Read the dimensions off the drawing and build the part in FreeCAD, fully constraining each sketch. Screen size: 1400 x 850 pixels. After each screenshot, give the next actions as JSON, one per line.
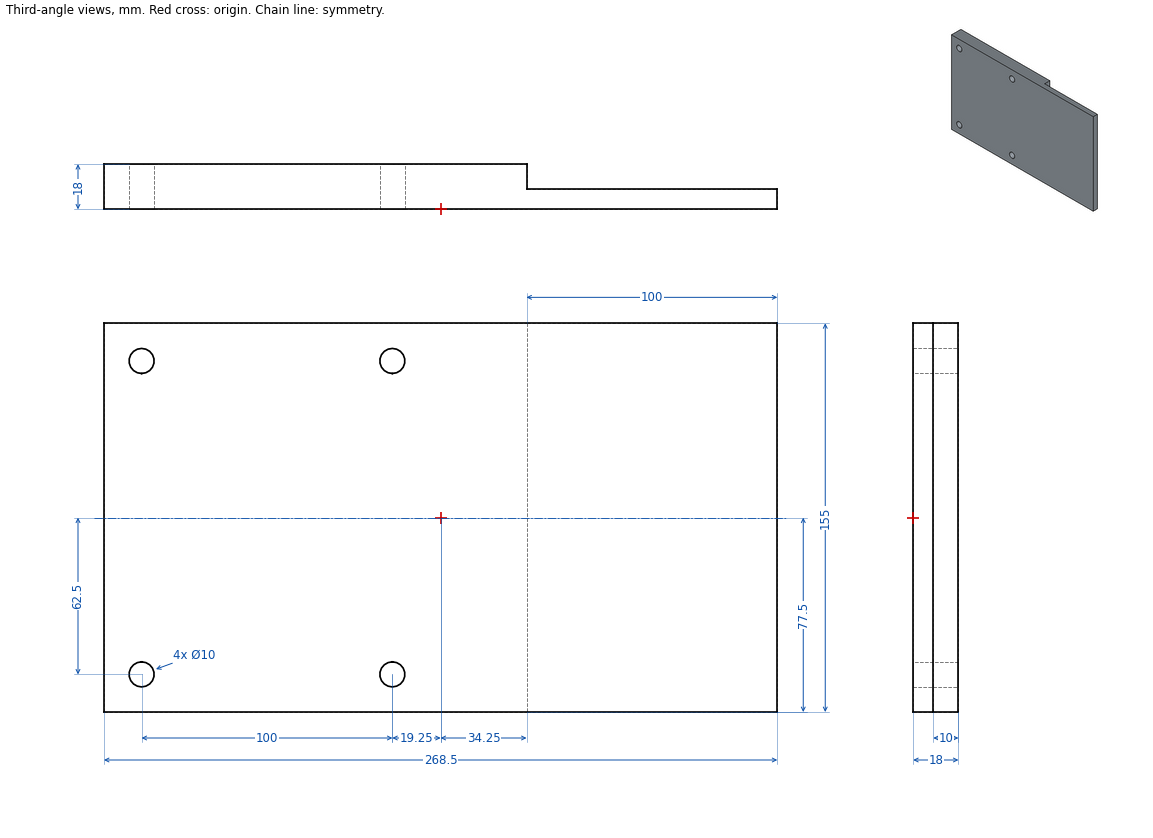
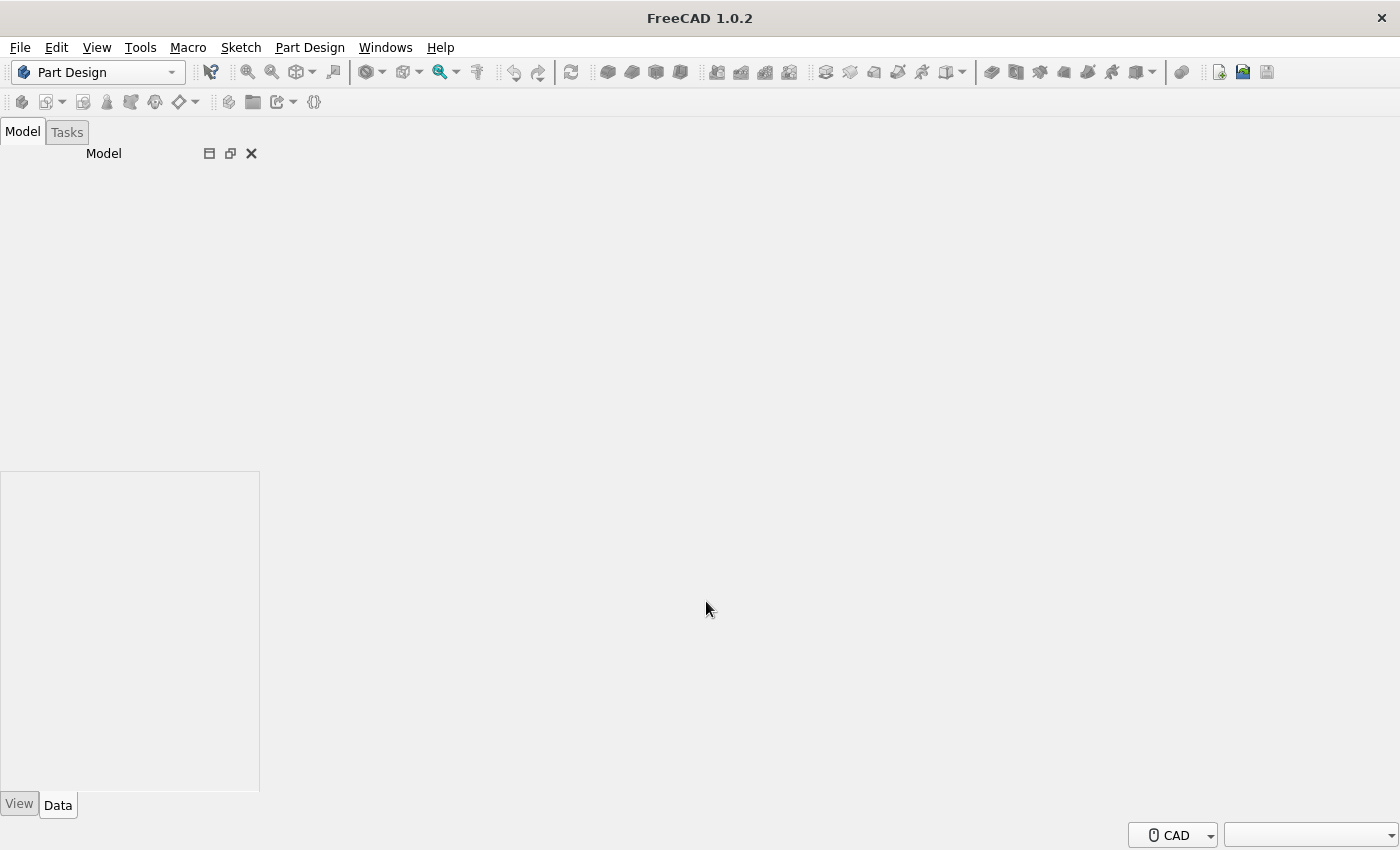
{"action": "left_click", "coordinate": [1220, 72]}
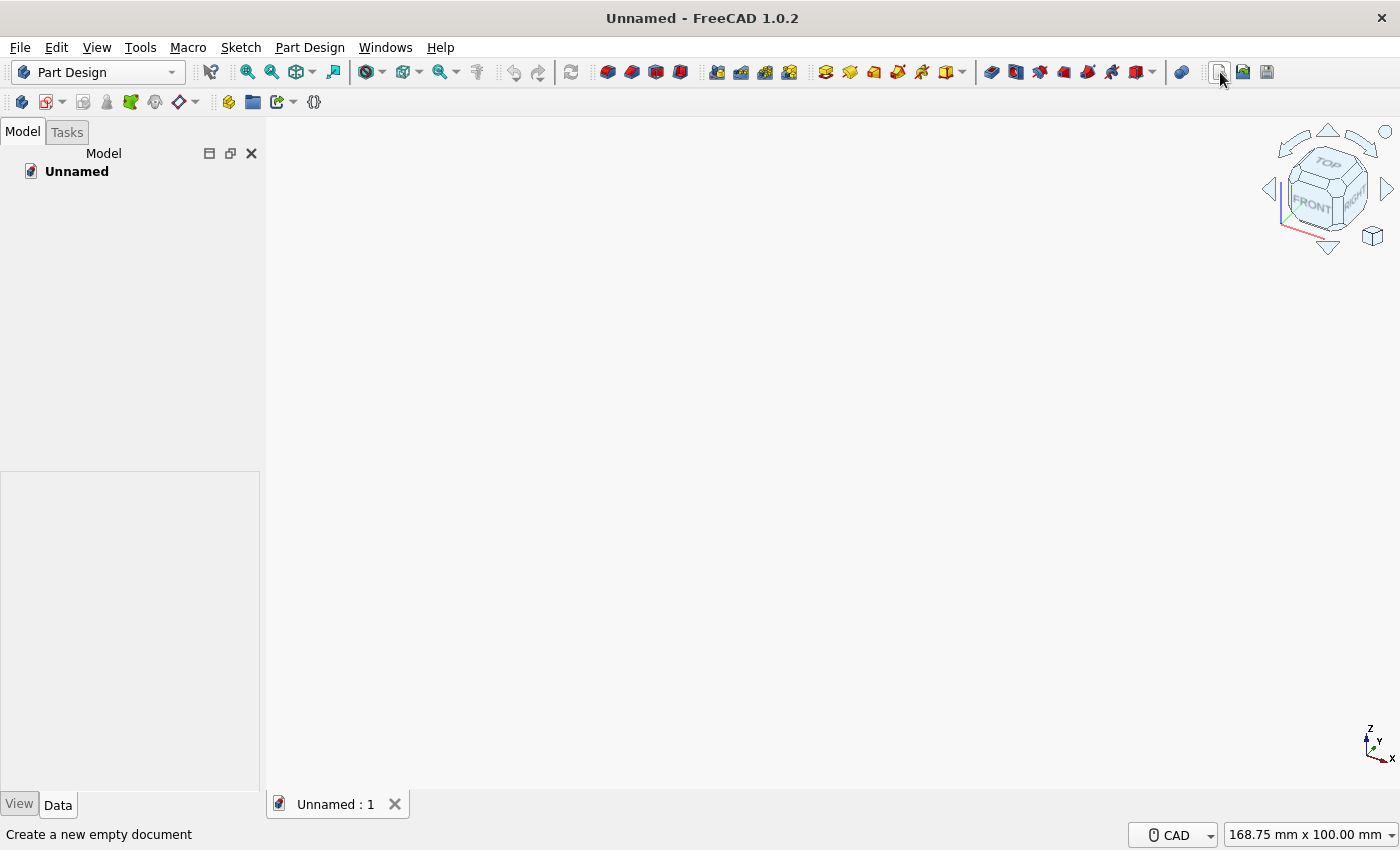
{"action": "left_click", "coordinate": [46, 102]}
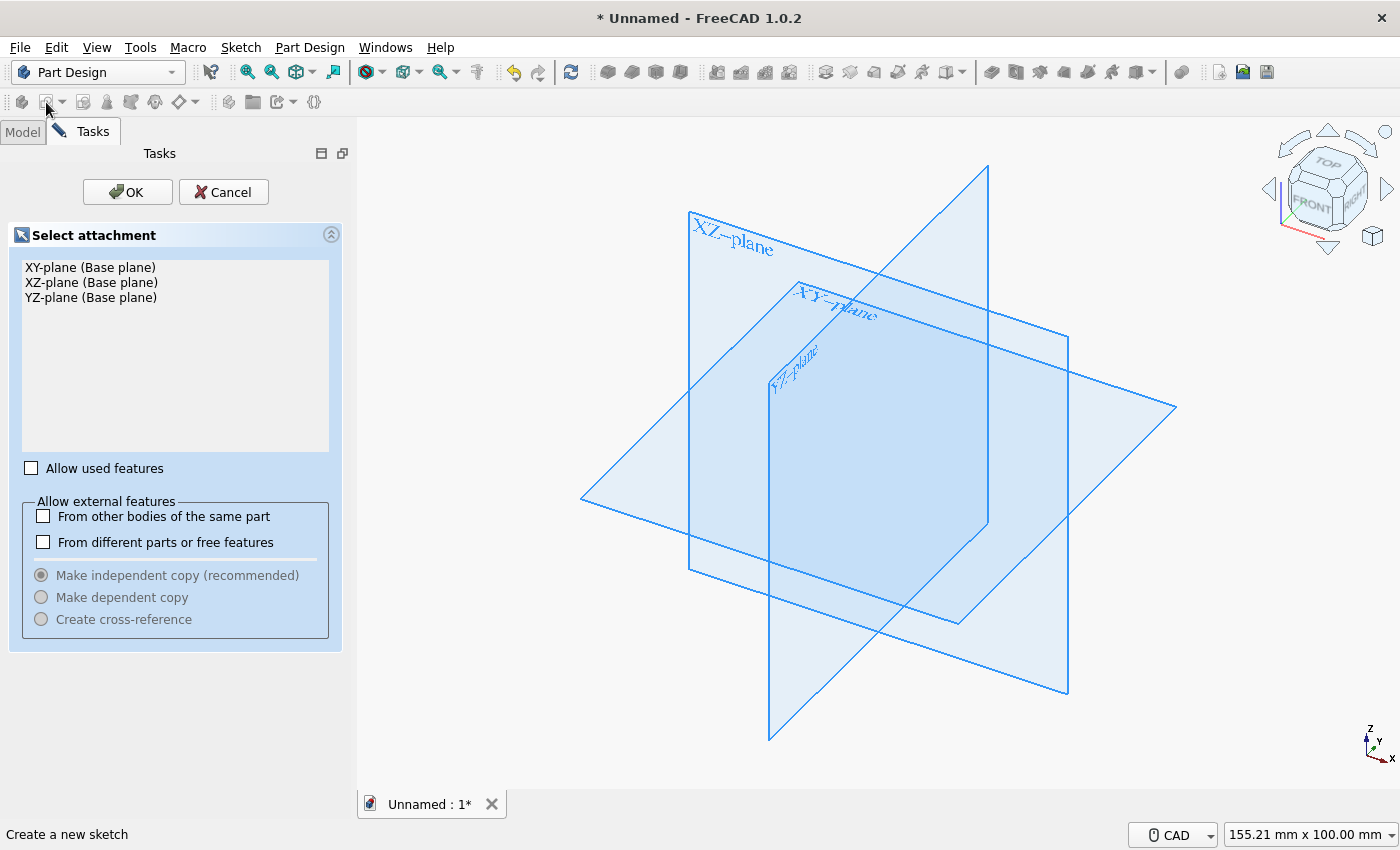
{"action": "left_click", "coordinate": [82, 282]}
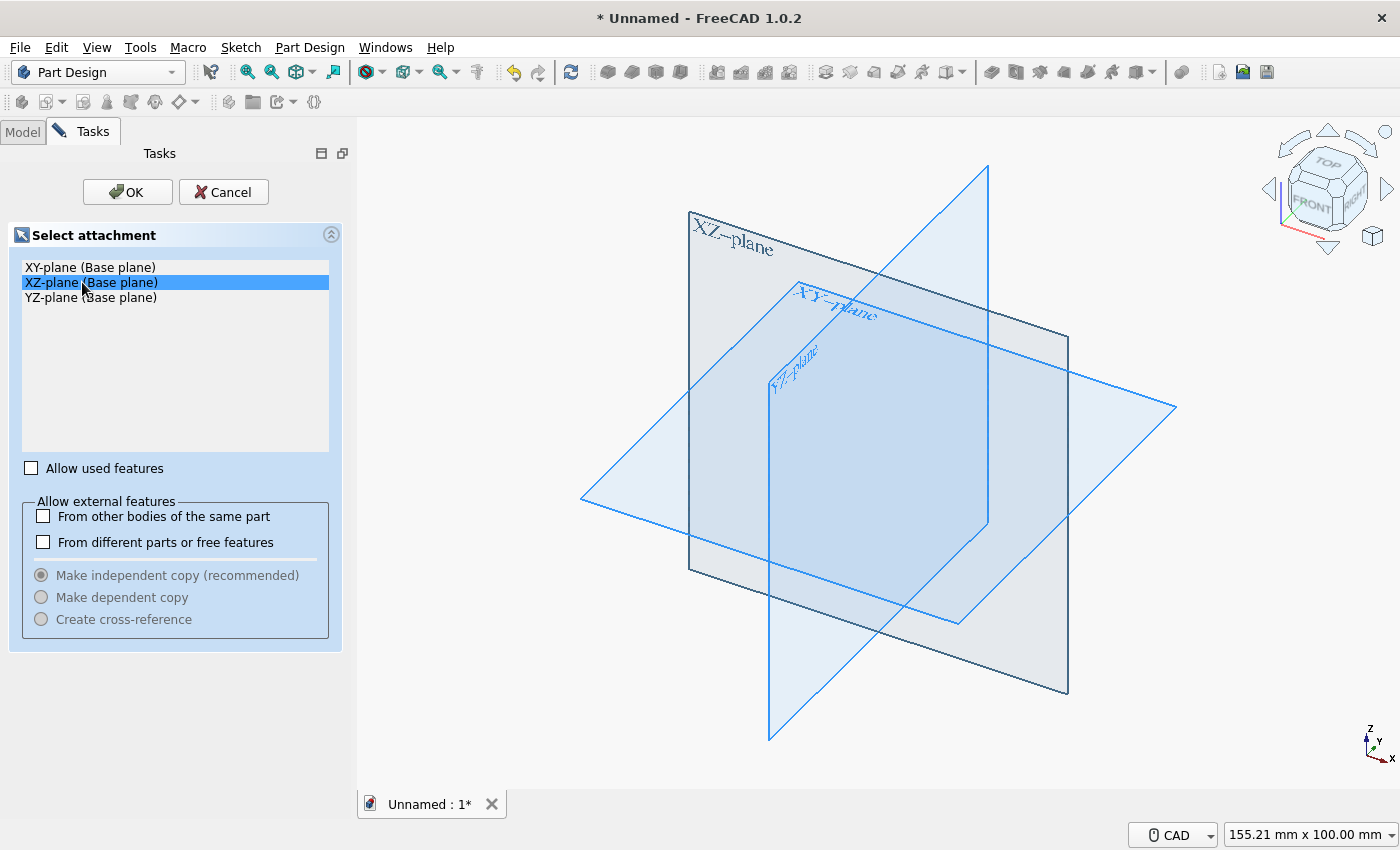
{"action": "left_click", "coordinate": [128, 192]}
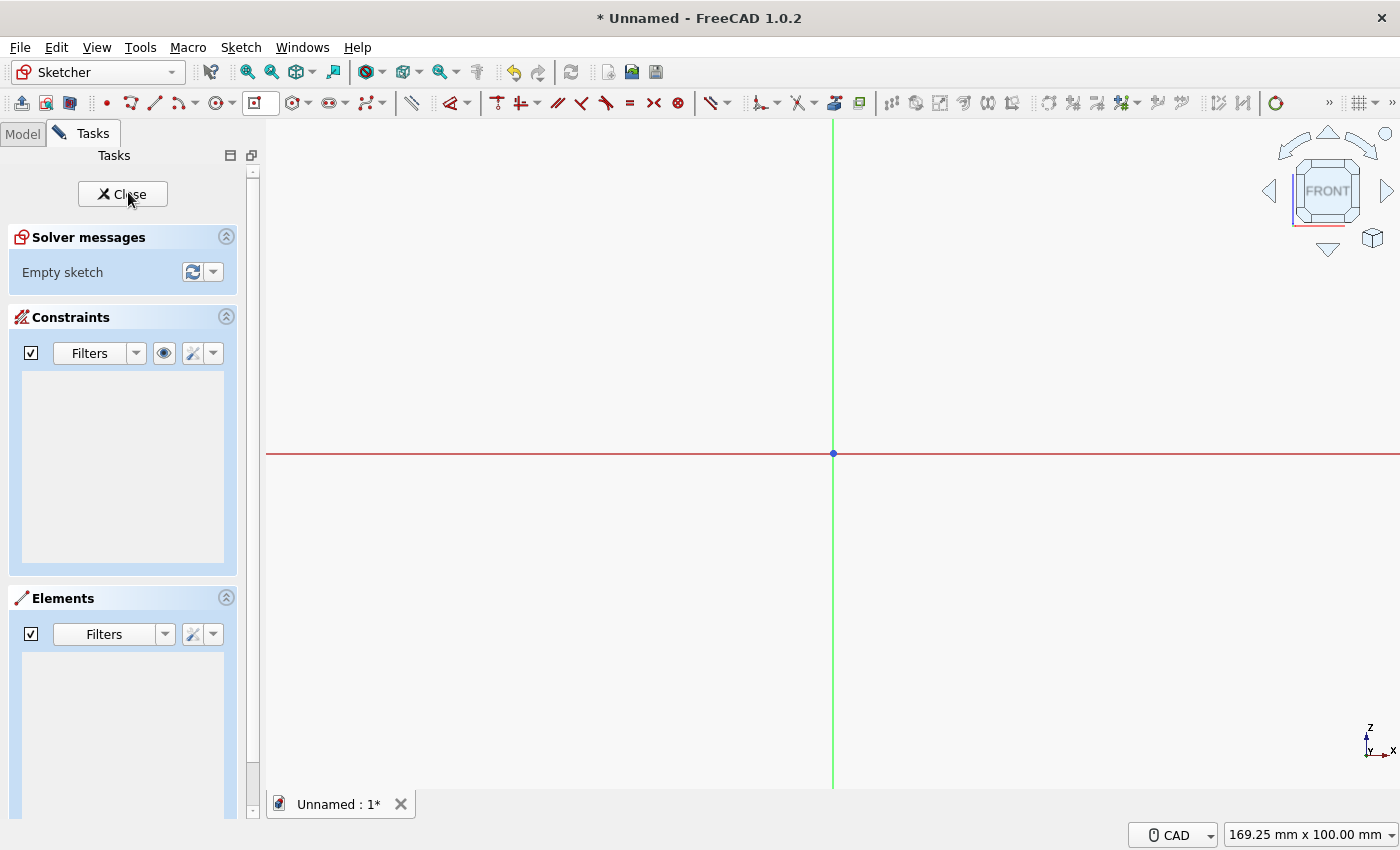
{"action": "scroll", "coordinate": [725, 454], "scroll_direction": "down", "scroll_amount": 5}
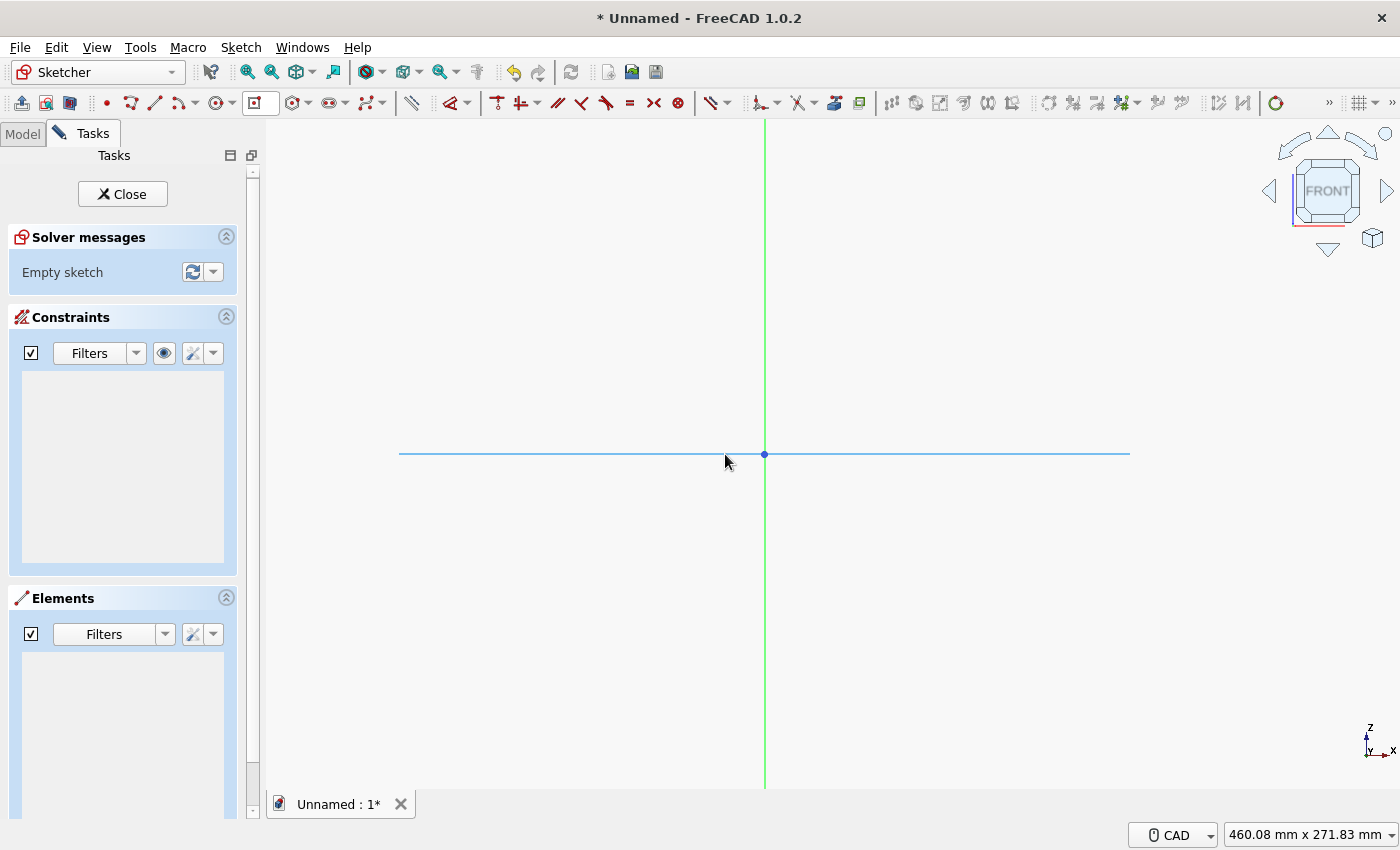
{"action": "key", "text": "g v"}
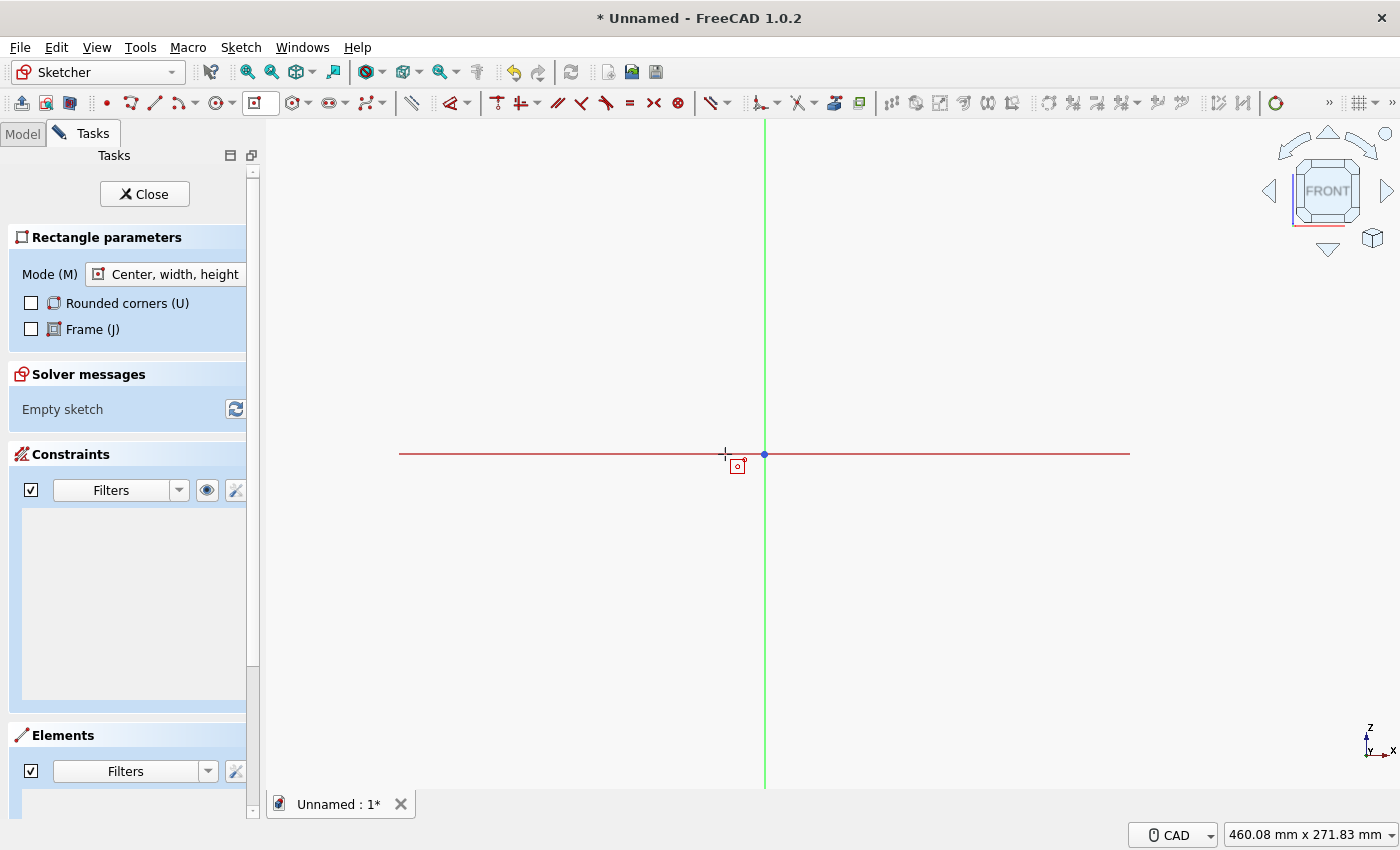
{"action": "left_click", "coordinate": [765, 454]}
{"action": "left_click", "coordinate": [1096, 263]}
{"action": "key", "text": "Escape"}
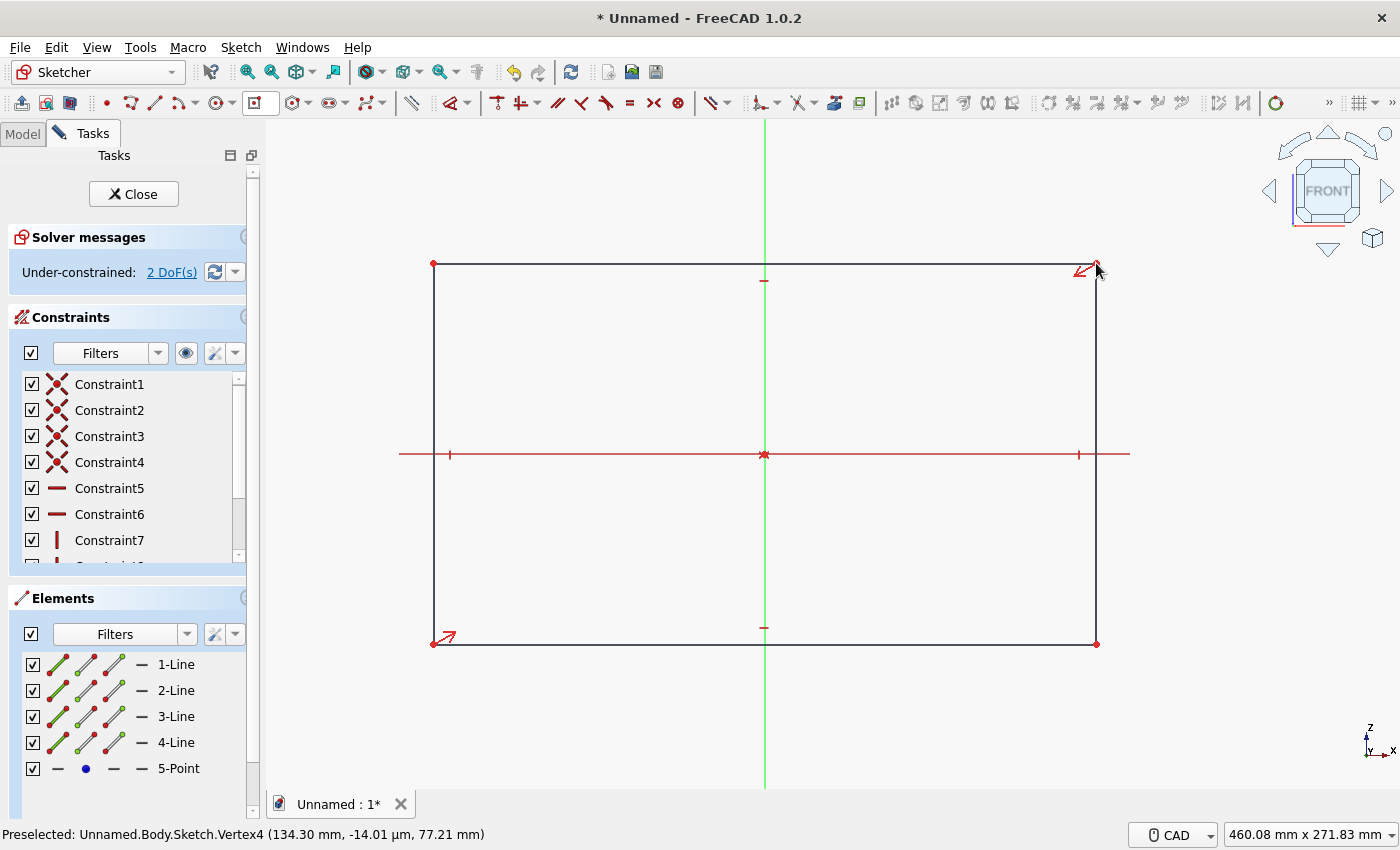
{"action": "left_click", "coordinate": [450, 104]}